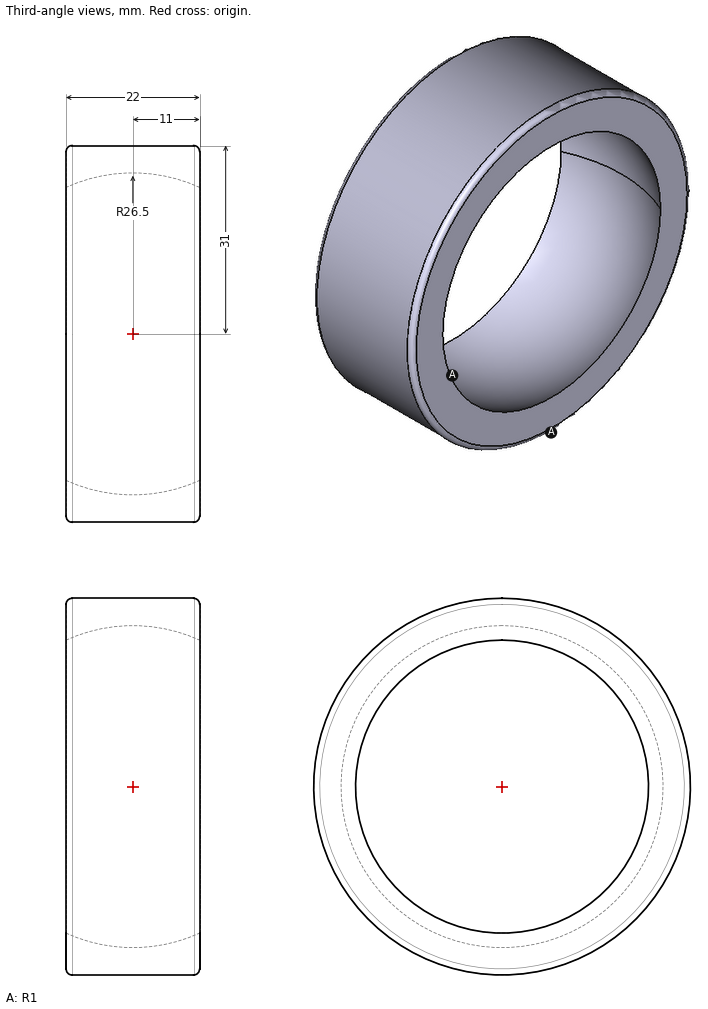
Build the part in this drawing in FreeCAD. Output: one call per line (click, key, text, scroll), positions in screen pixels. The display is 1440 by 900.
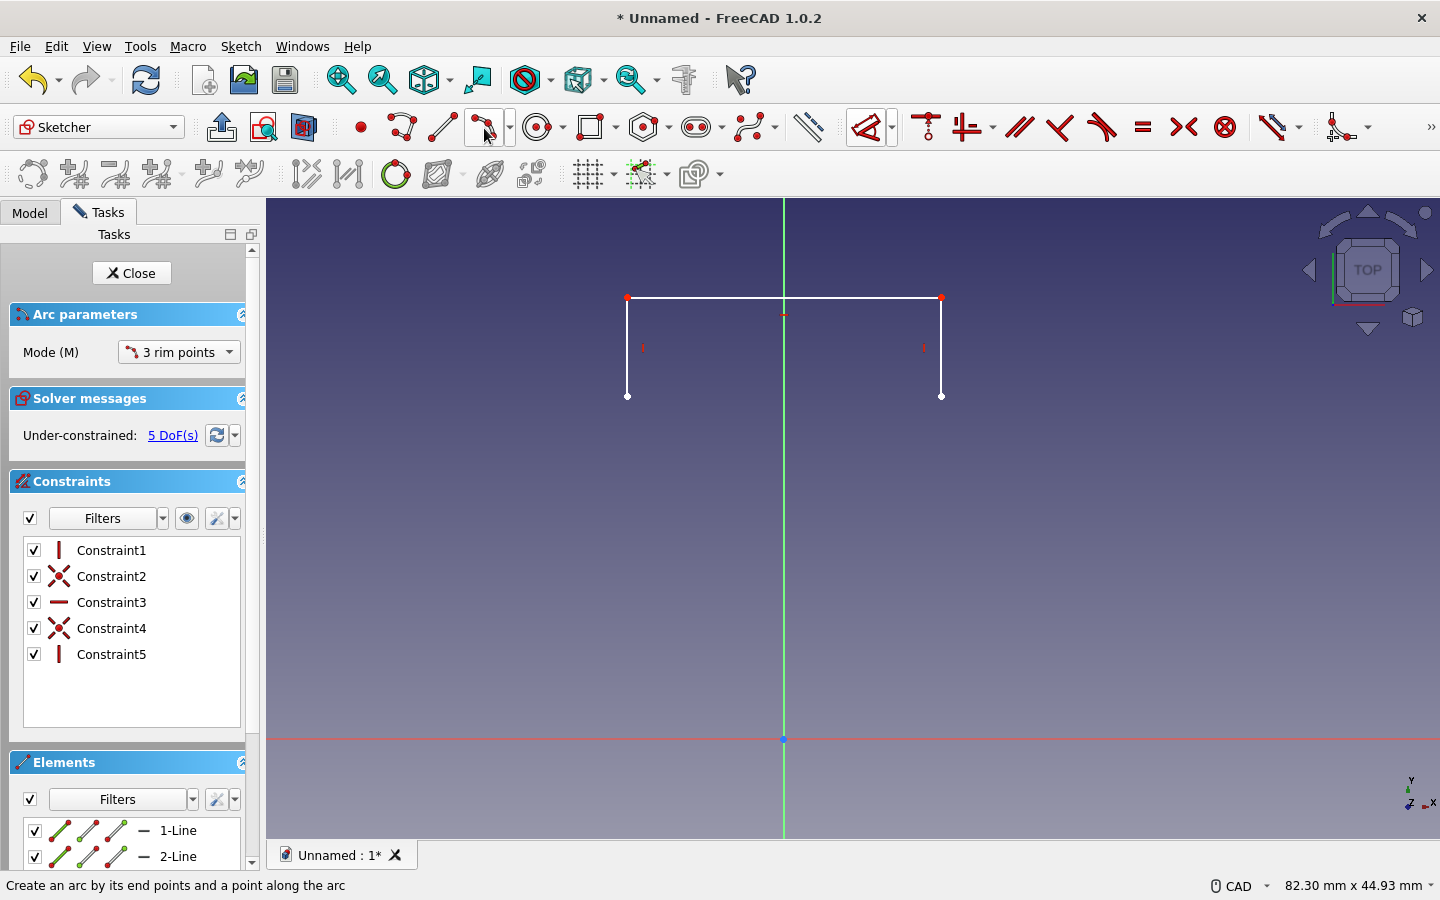
click(627, 397)
click(941, 397)
click(816, 363)
key(Escape)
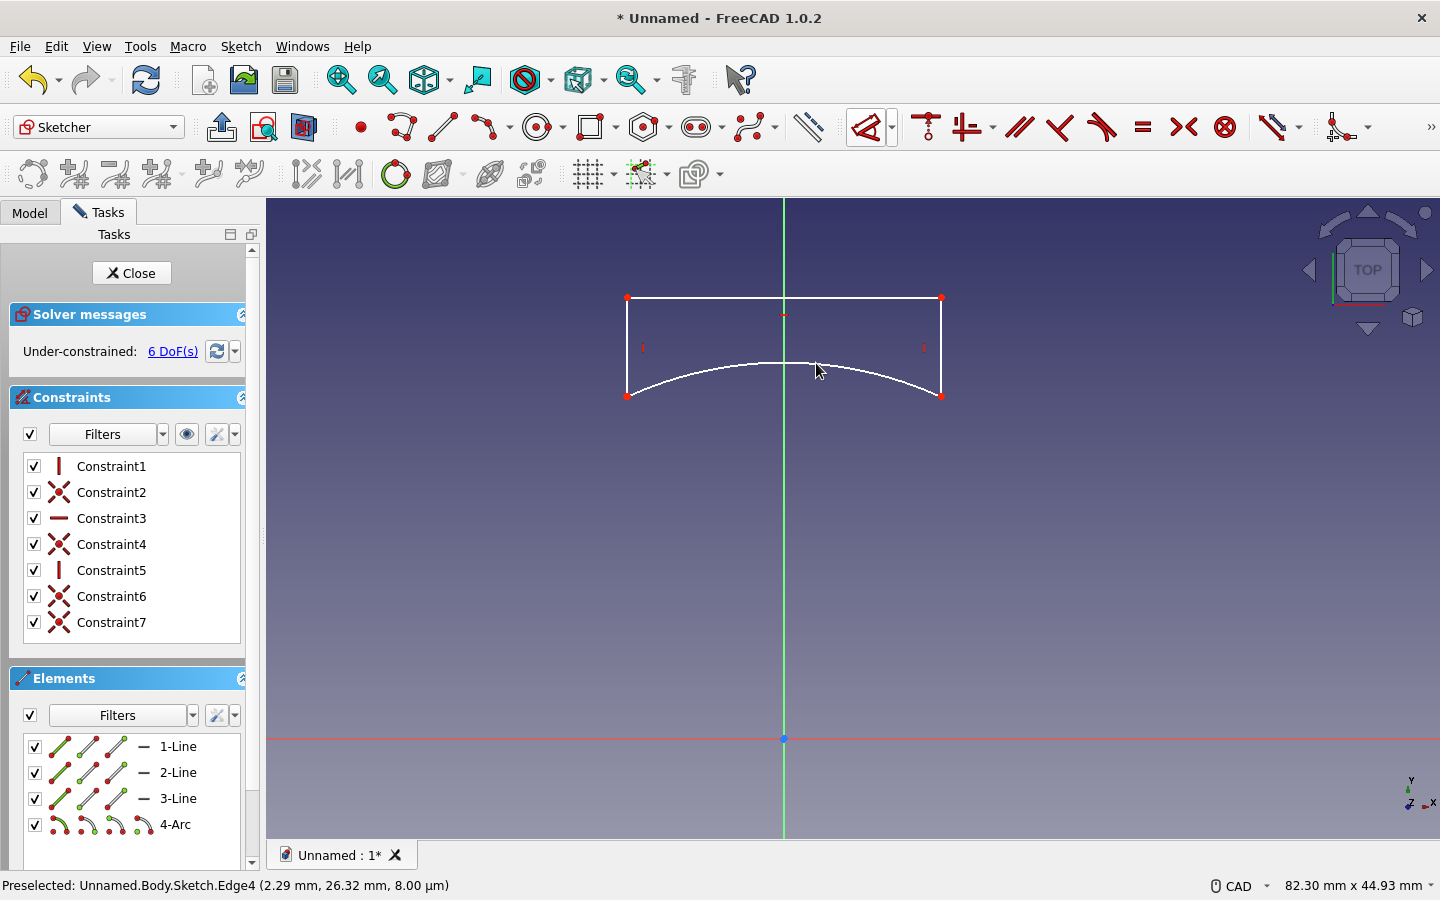
drag(774, 728, 794, 749)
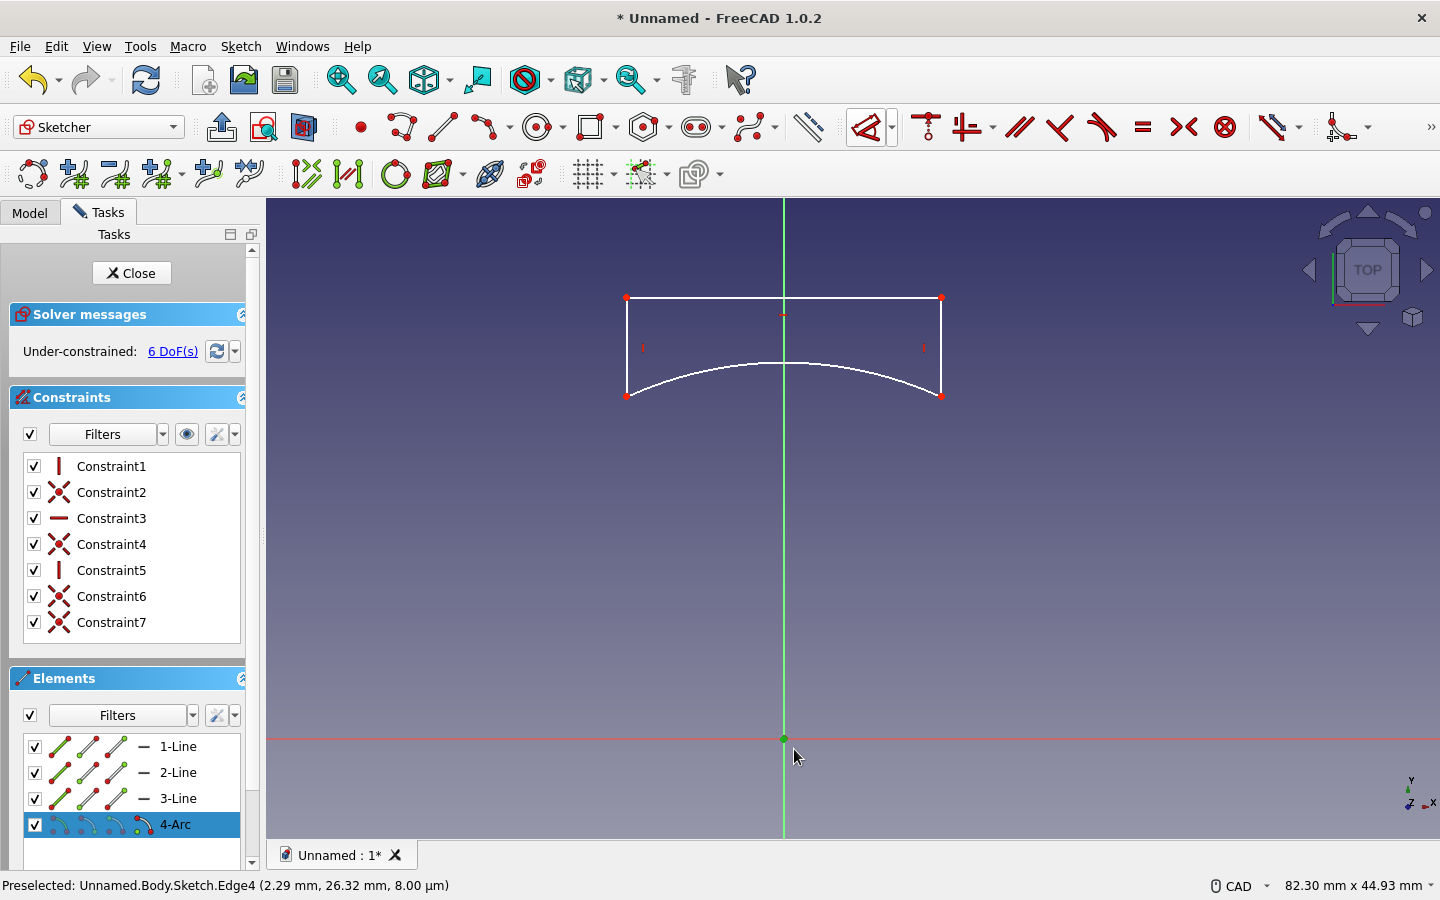
click(926, 128)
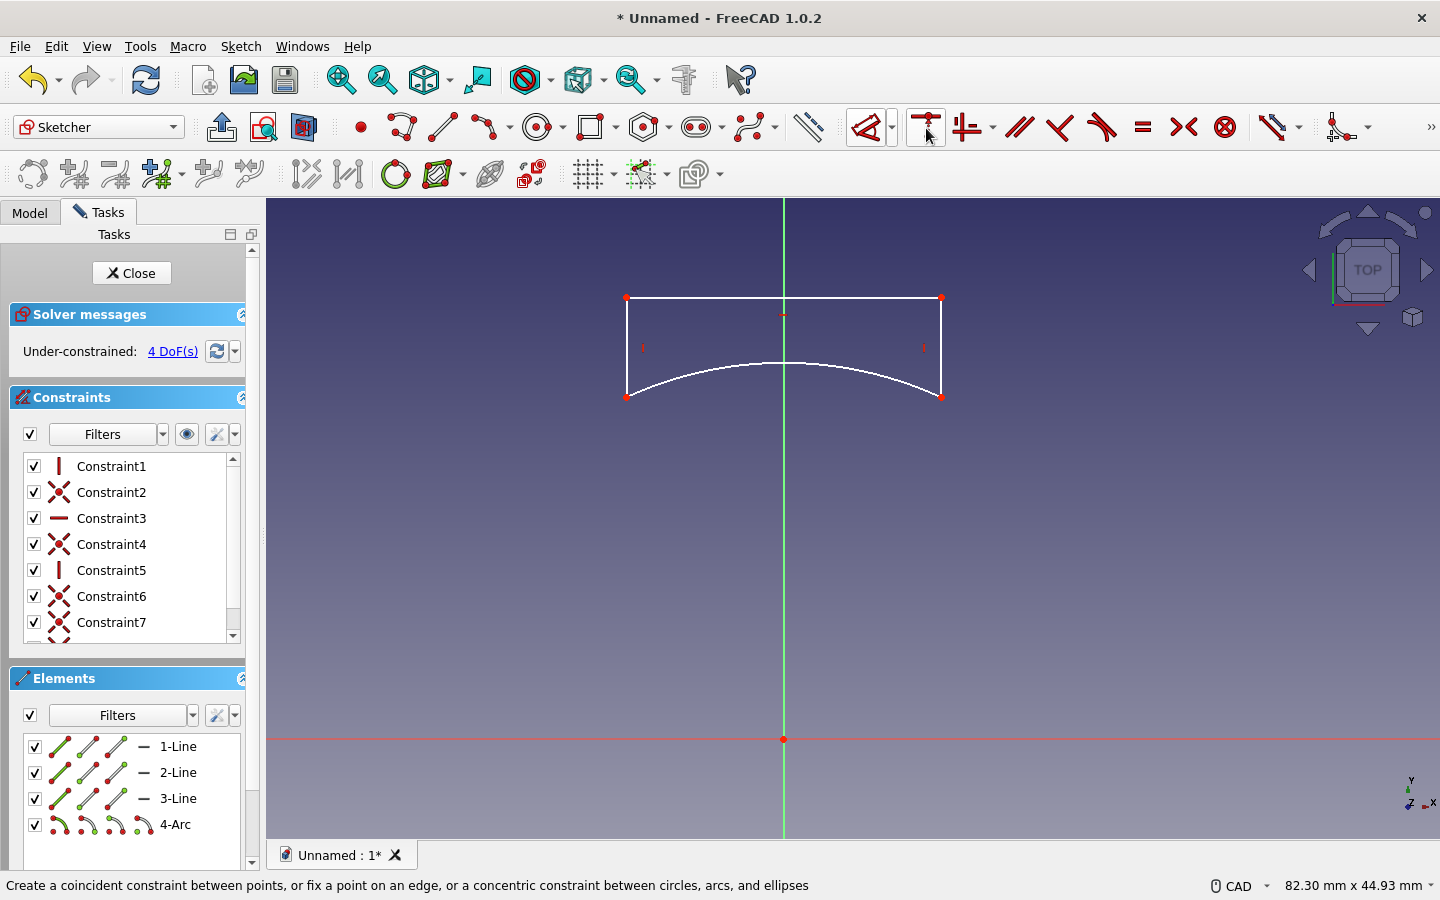
click(866, 128)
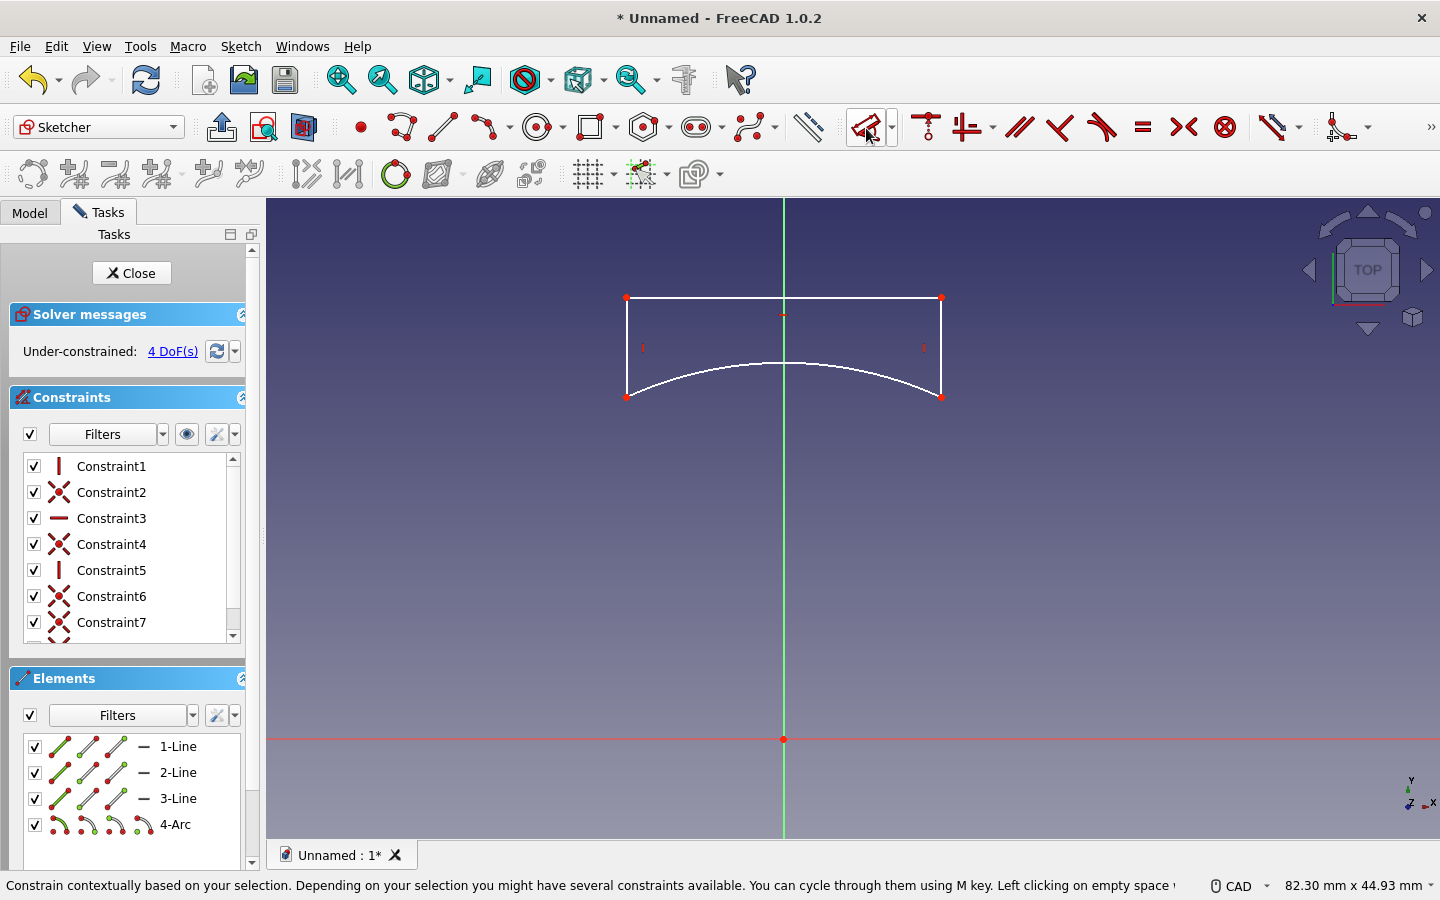
click(848, 368)
click(853, 336)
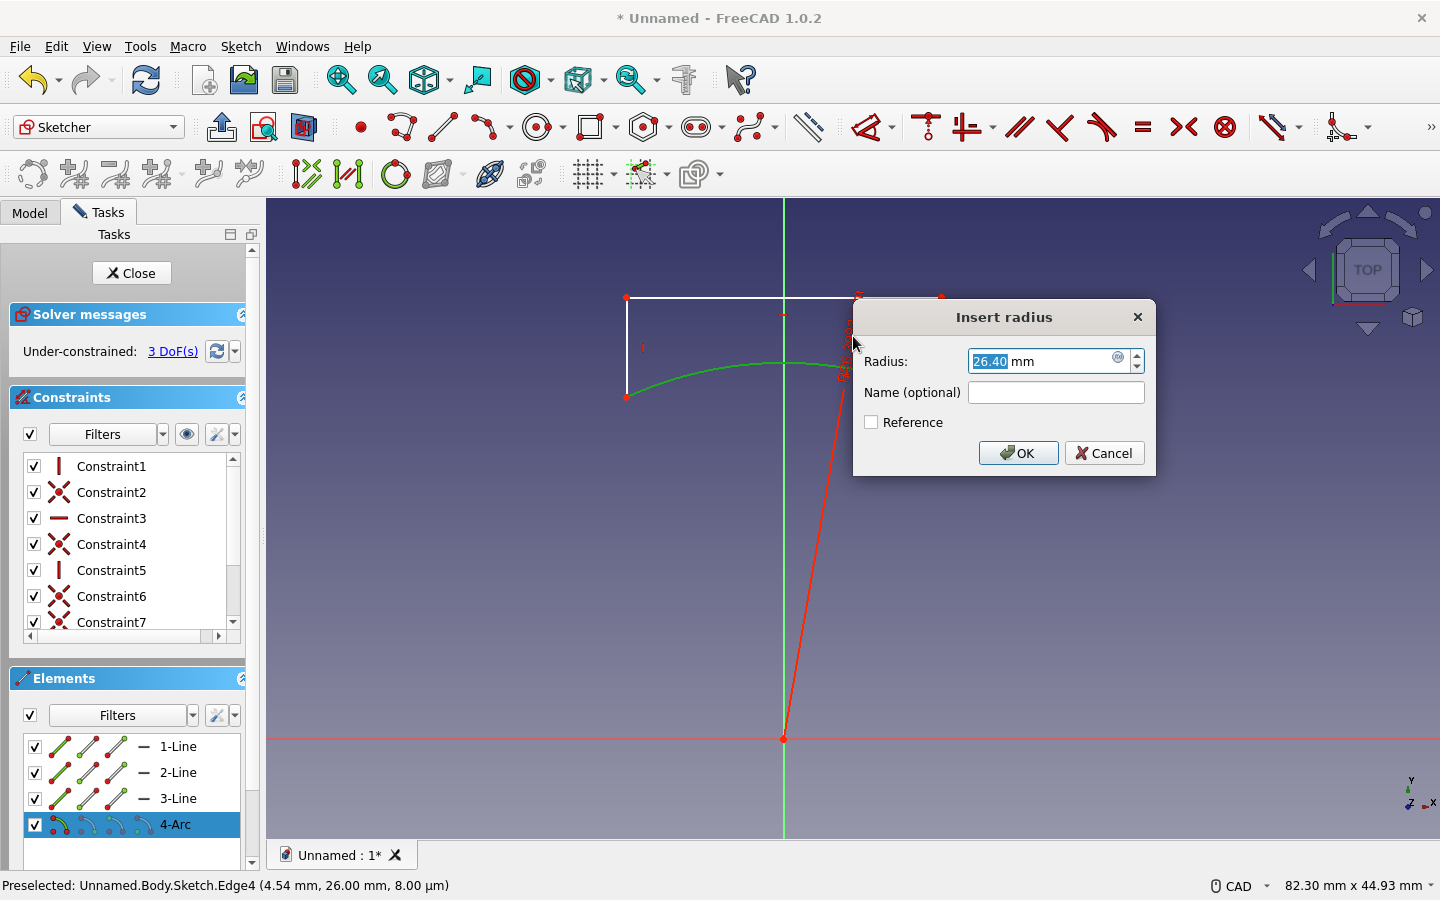
text(26.5)
key(Return)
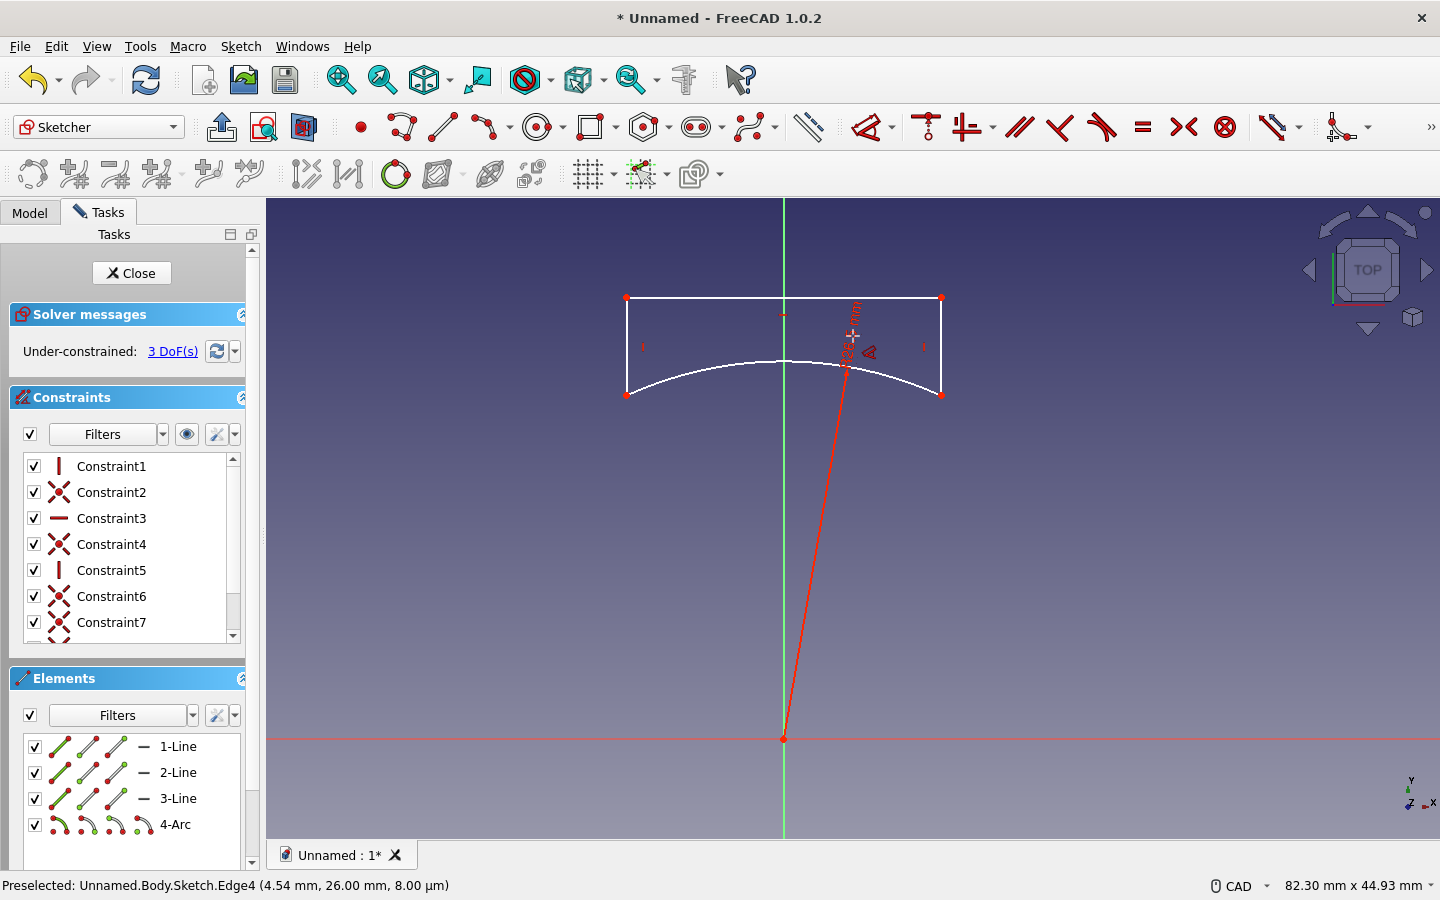
click(847, 298)
click(712, 264)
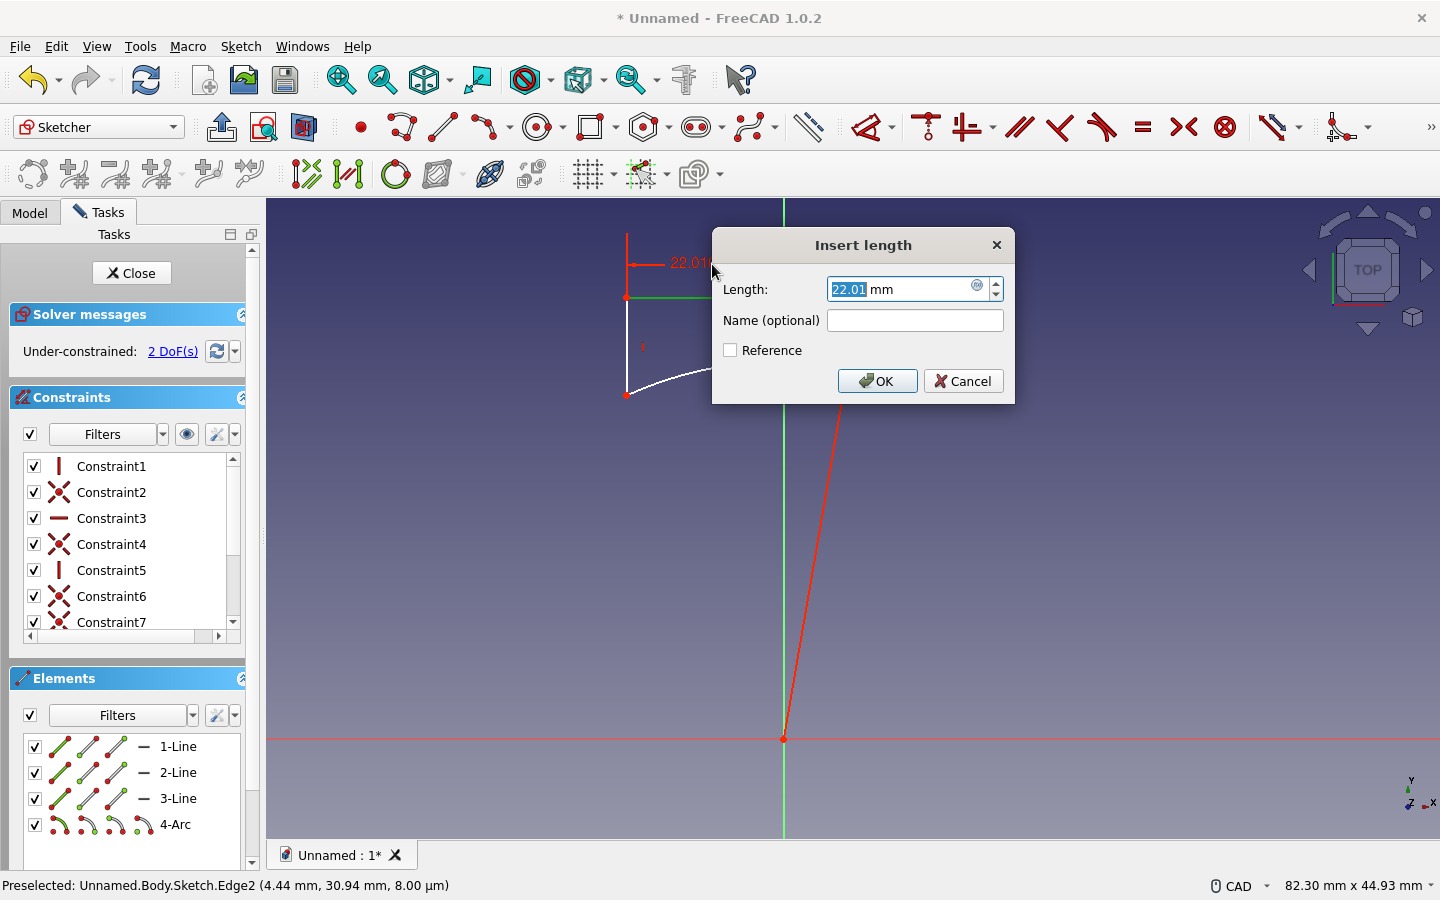
text(22)
key(Return)